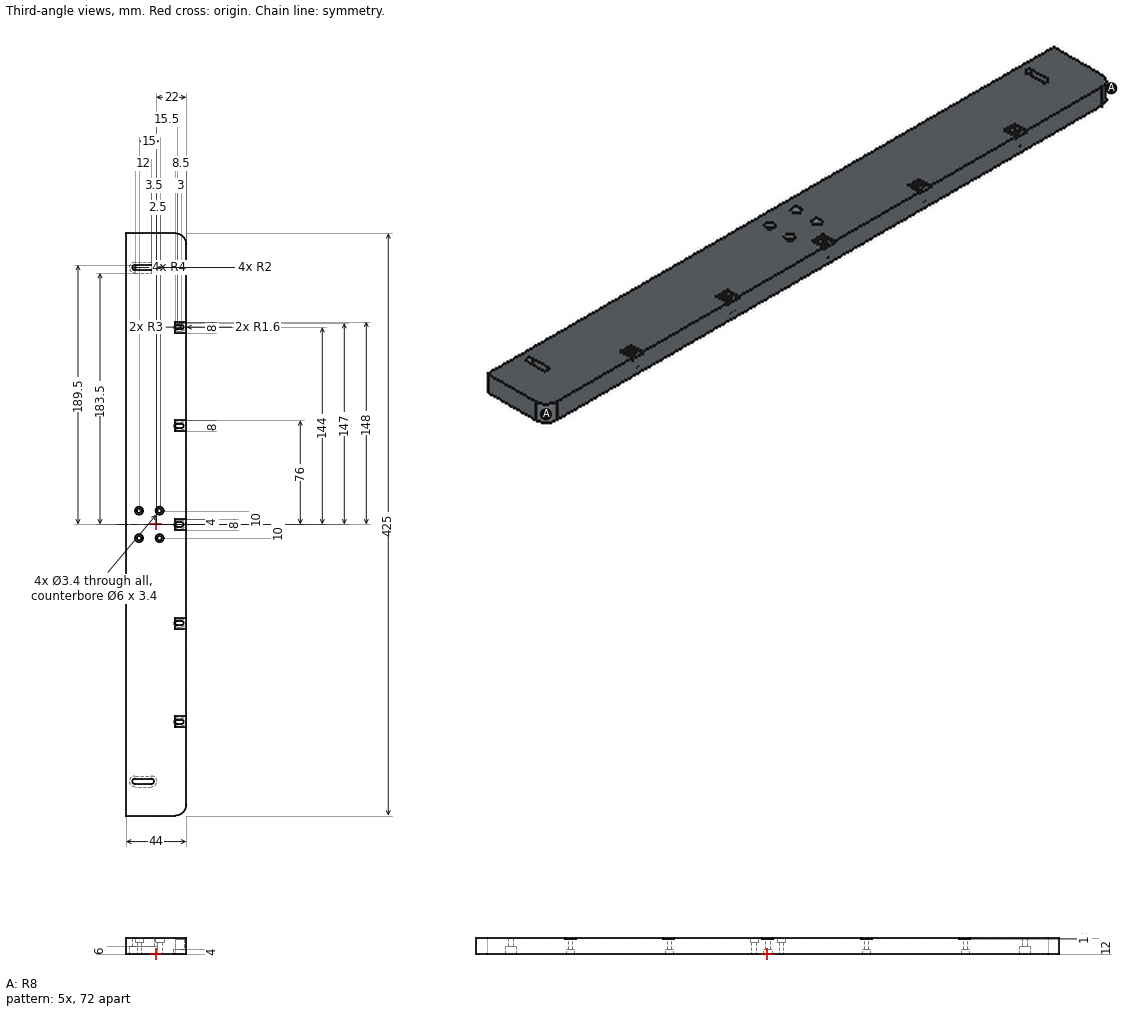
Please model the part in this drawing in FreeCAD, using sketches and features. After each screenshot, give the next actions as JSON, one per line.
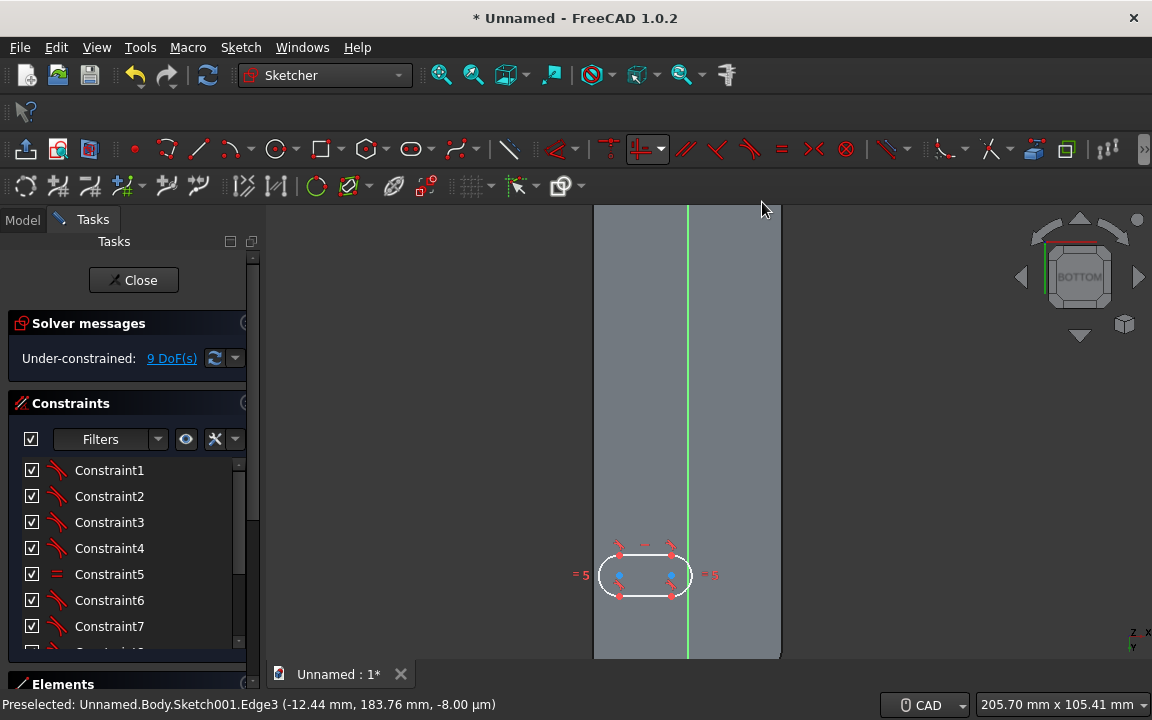
{"action": "scroll", "coordinate": [639, 564], "scroll_direction": "down", "scroll_amount": 9}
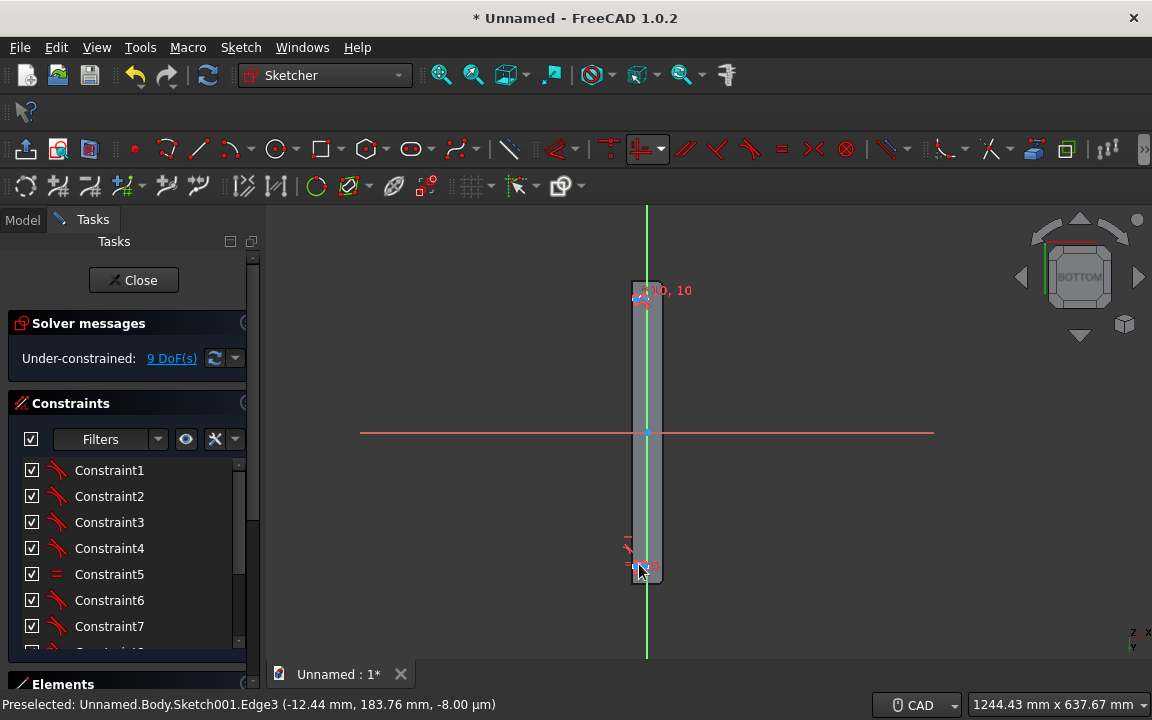
{"action": "scroll", "coordinate": [639, 297], "scroll_direction": "up", "scroll_amount": 9}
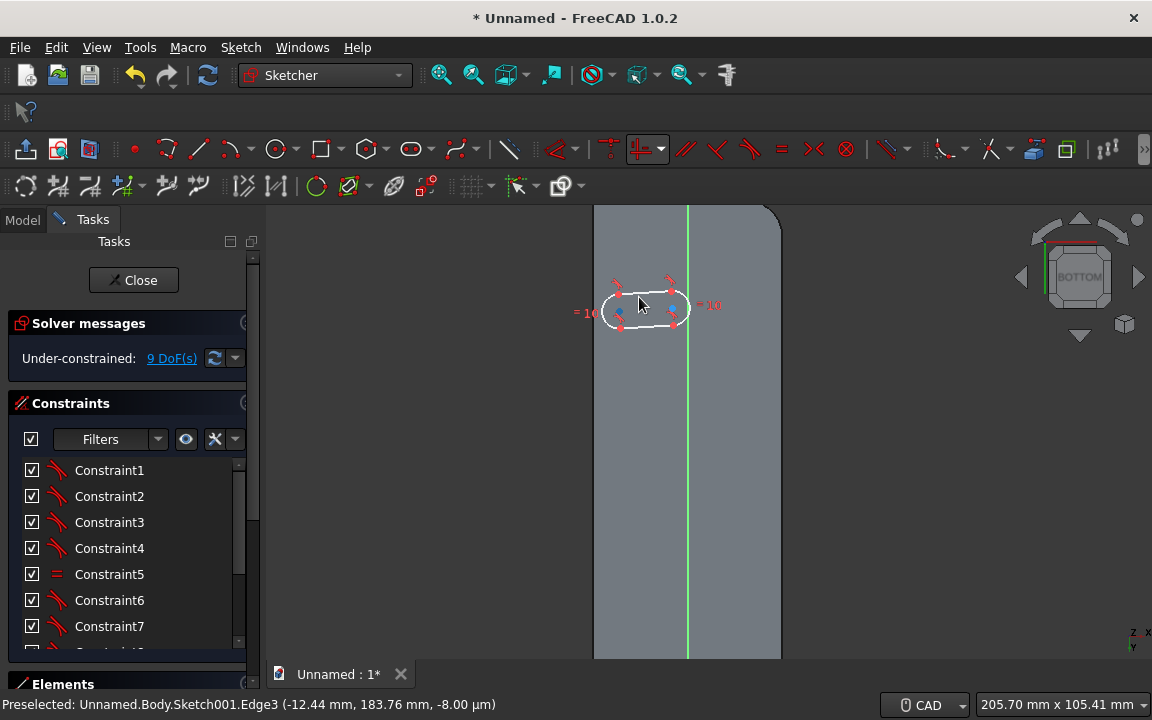
{"action": "left_click", "coordinate": [634, 293]}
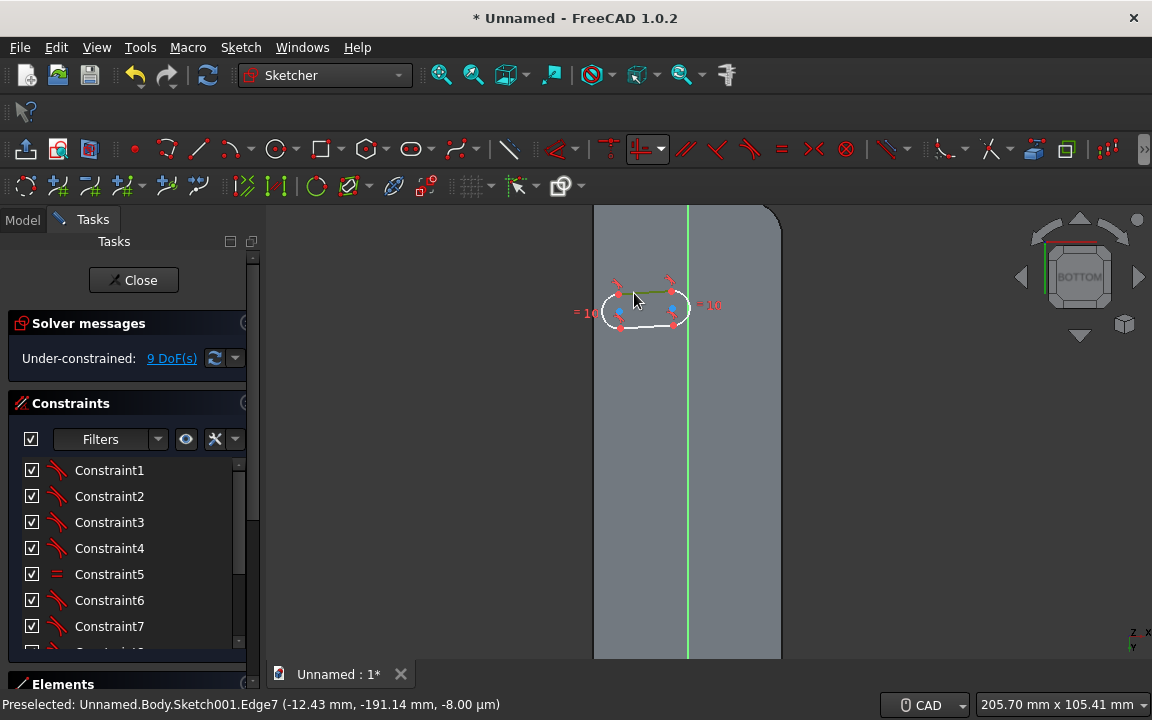
{"action": "key", "text": "h"}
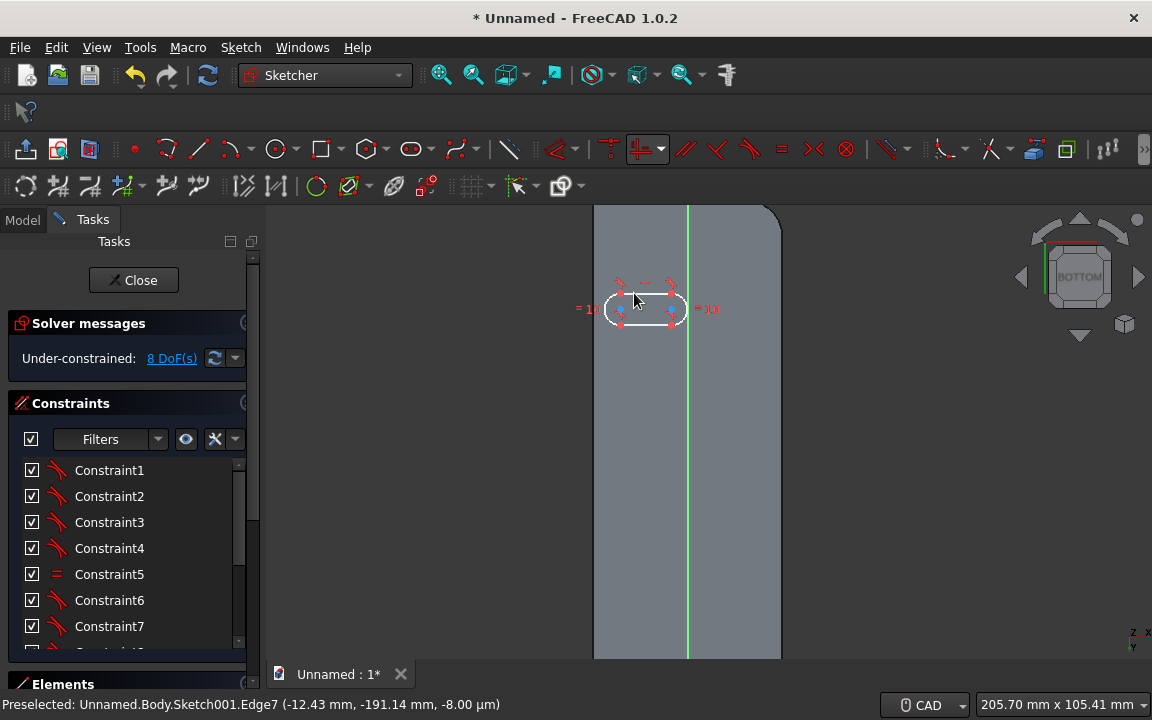
{"action": "scroll", "coordinate": [639, 296], "scroll_direction": "down", "scroll_amount": 9}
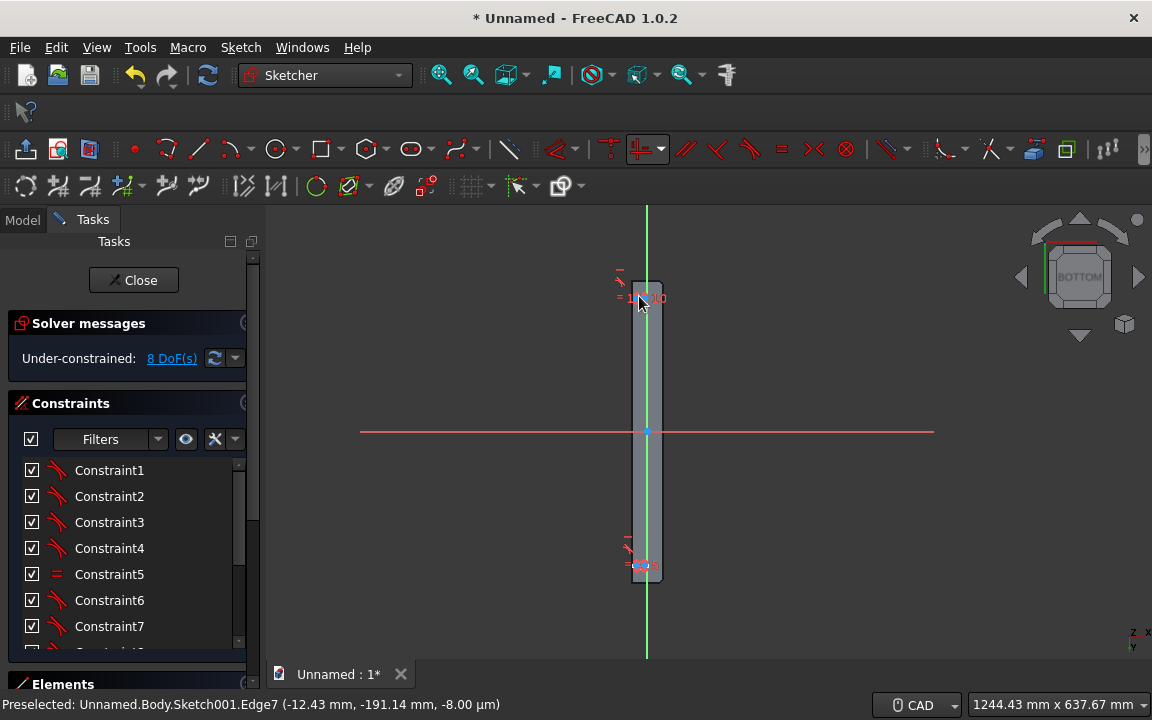
{"action": "scroll", "coordinate": [633, 564], "scroll_direction": "up", "scroll_amount": 8}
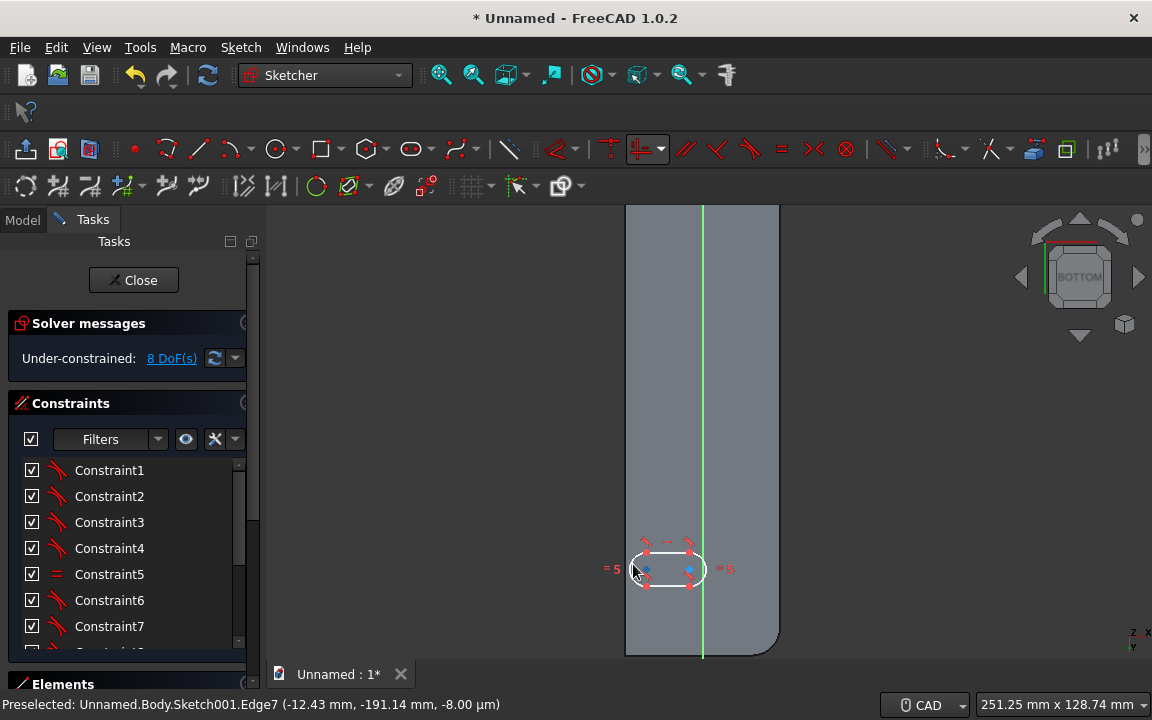
{"action": "left_click", "coordinate": [633, 560]}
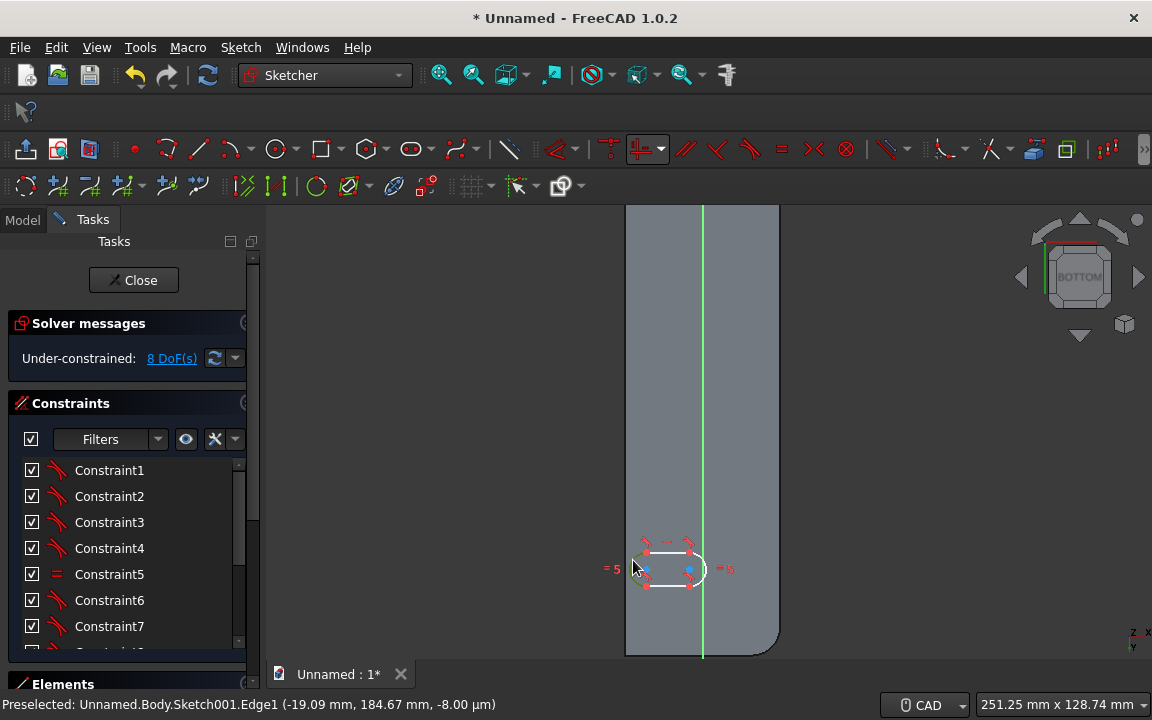
{"action": "scroll", "coordinate": [633, 565], "scroll_direction": "down", "scroll_amount": 8}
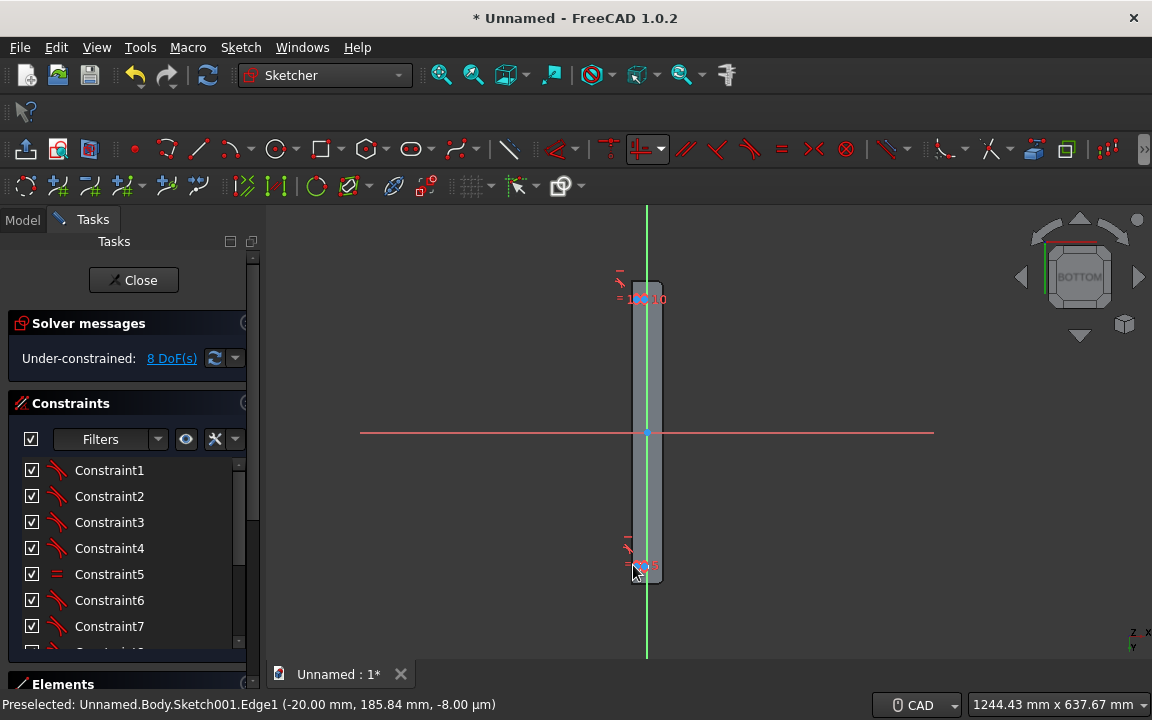
{"action": "scroll", "coordinate": [634, 298], "scroll_direction": "up", "scroll_amount": 9}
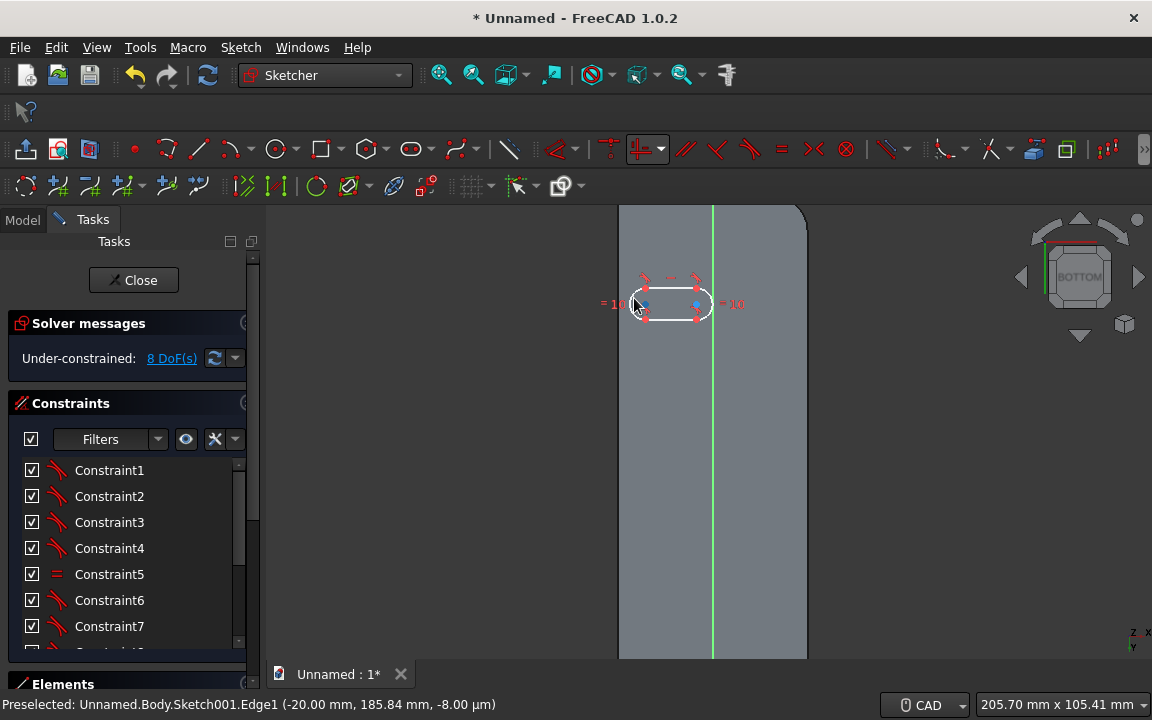
{"action": "left_click", "coordinate": [633, 295]}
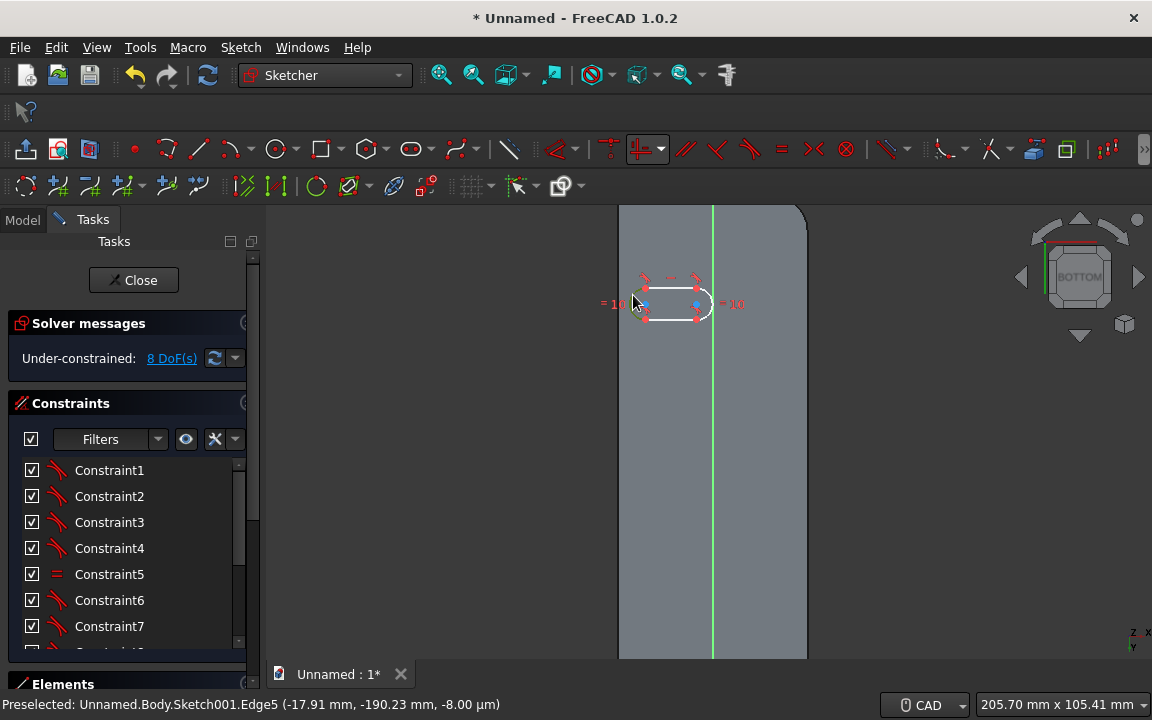
{"action": "key", "text": "e"}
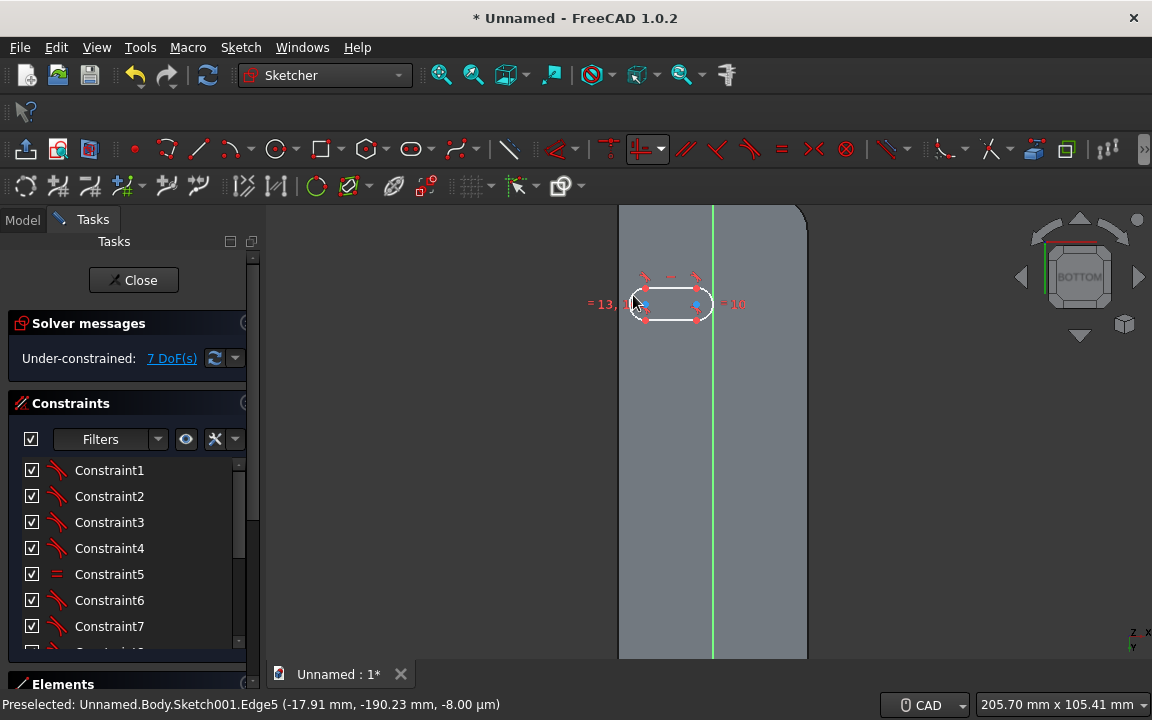
{"action": "scroll", "coordinate": [634, 297], "scroll_direction": "down", "scroll_amount": 9}